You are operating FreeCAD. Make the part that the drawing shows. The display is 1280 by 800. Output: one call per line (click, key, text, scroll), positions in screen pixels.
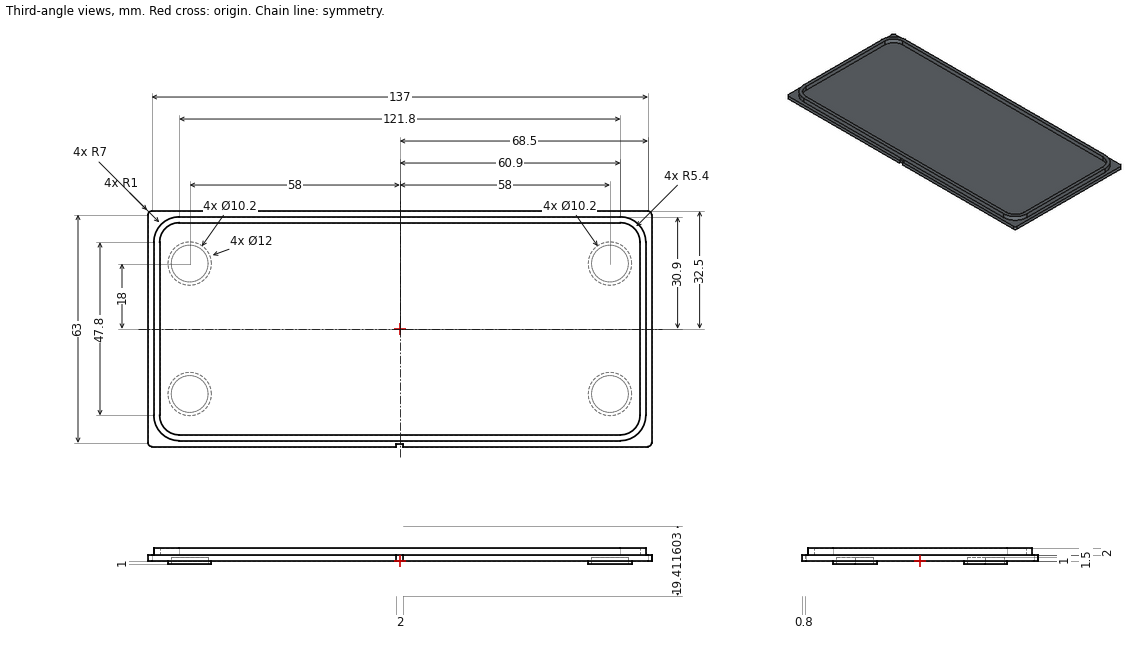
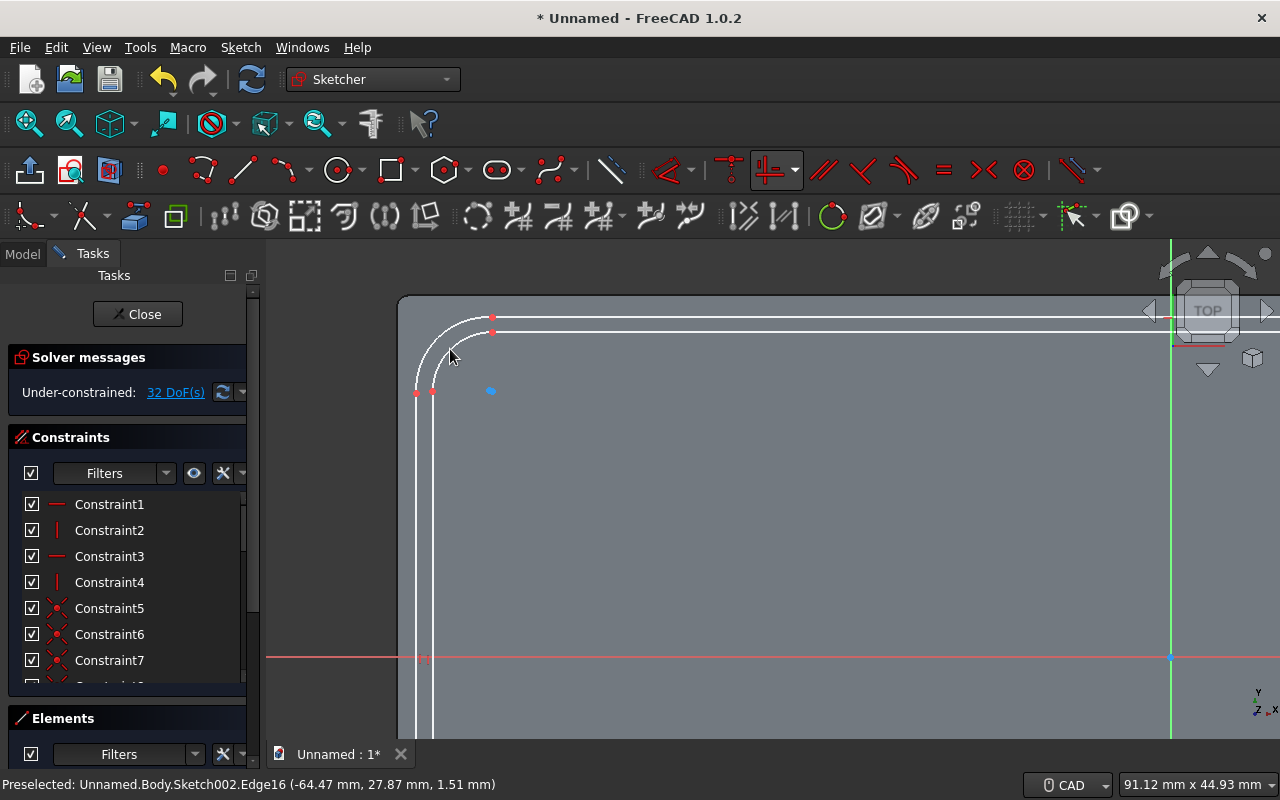
click(899, 317)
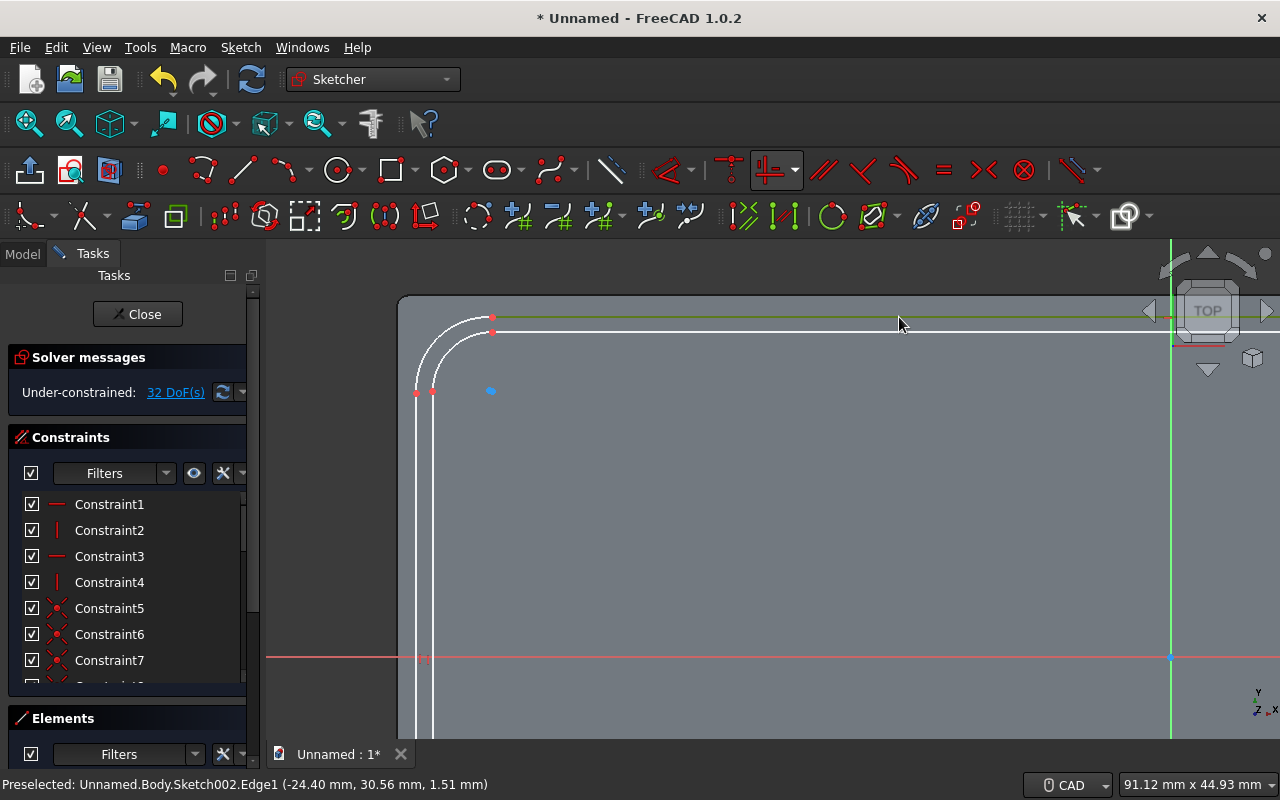
click(457, 324)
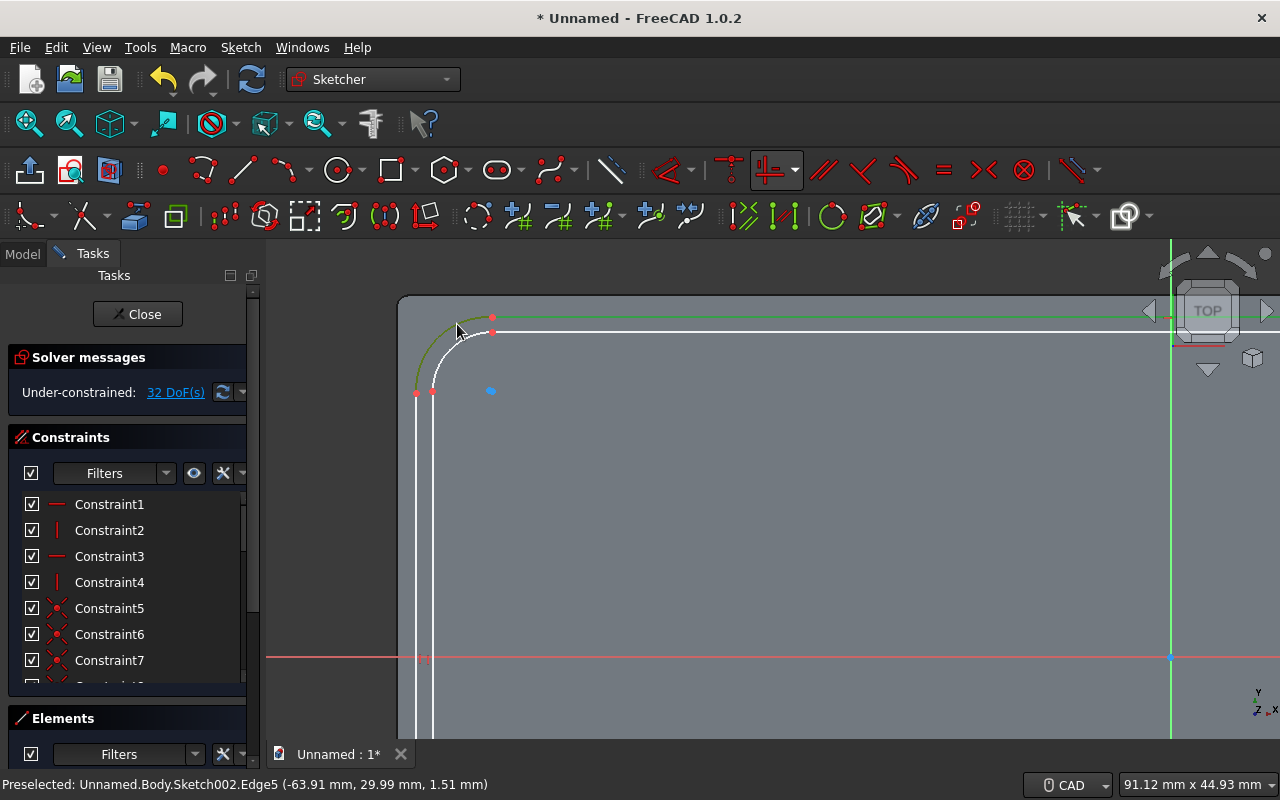
click(904, 170)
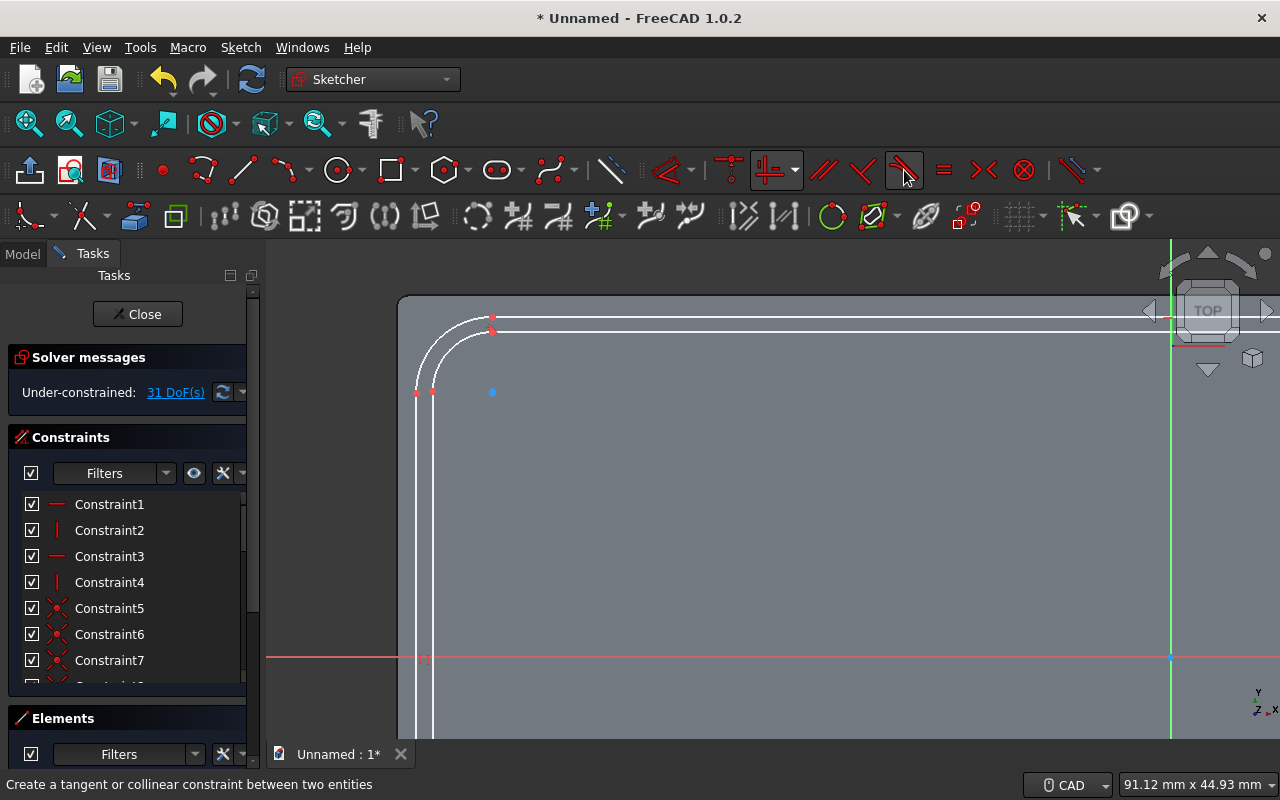
click(899, 317)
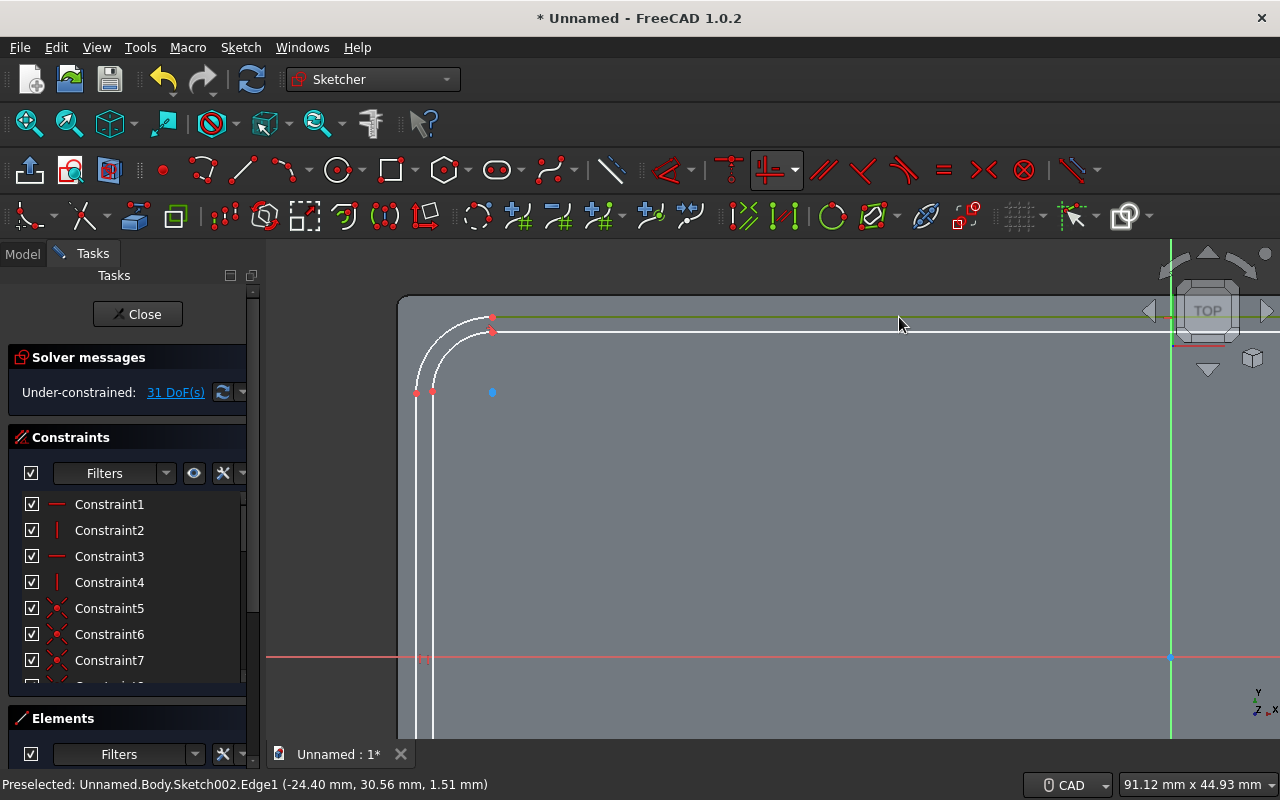
scroll(433, 391, down, 5)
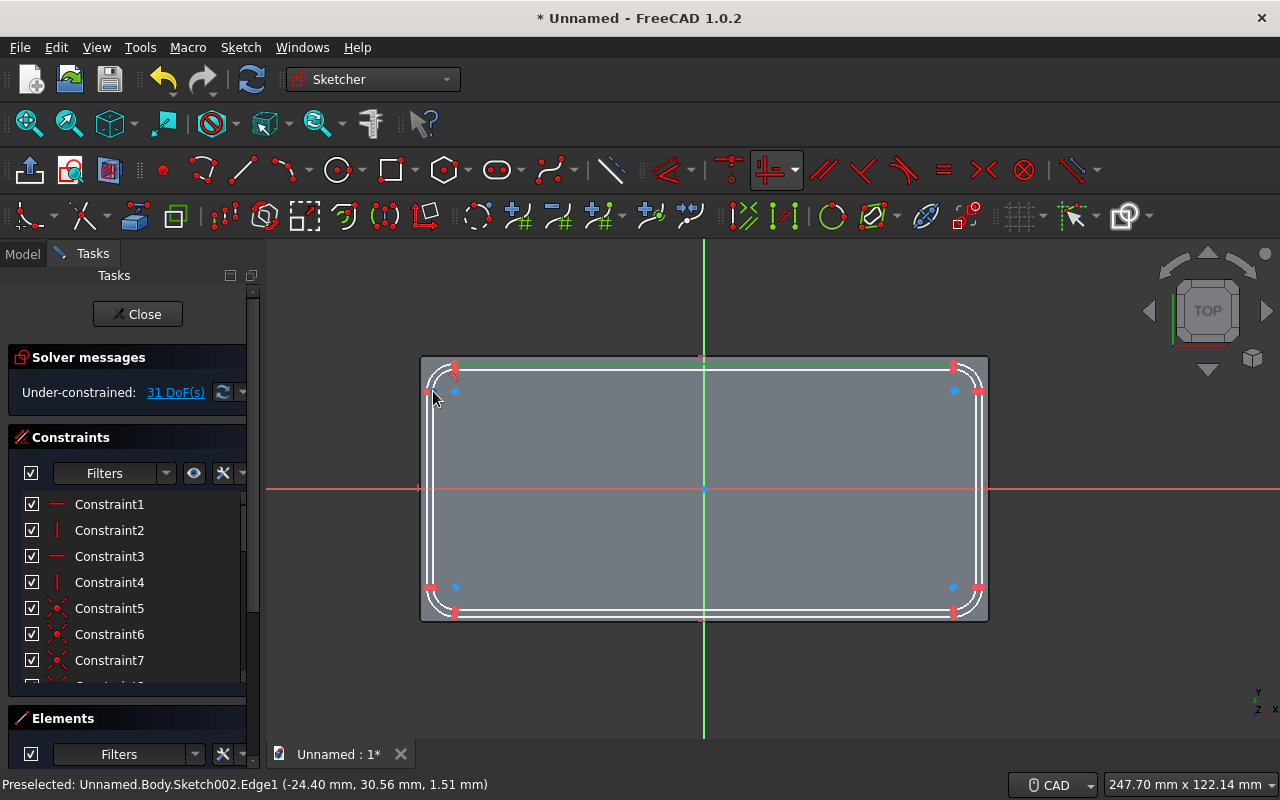
scroll(979, 379, up, 4)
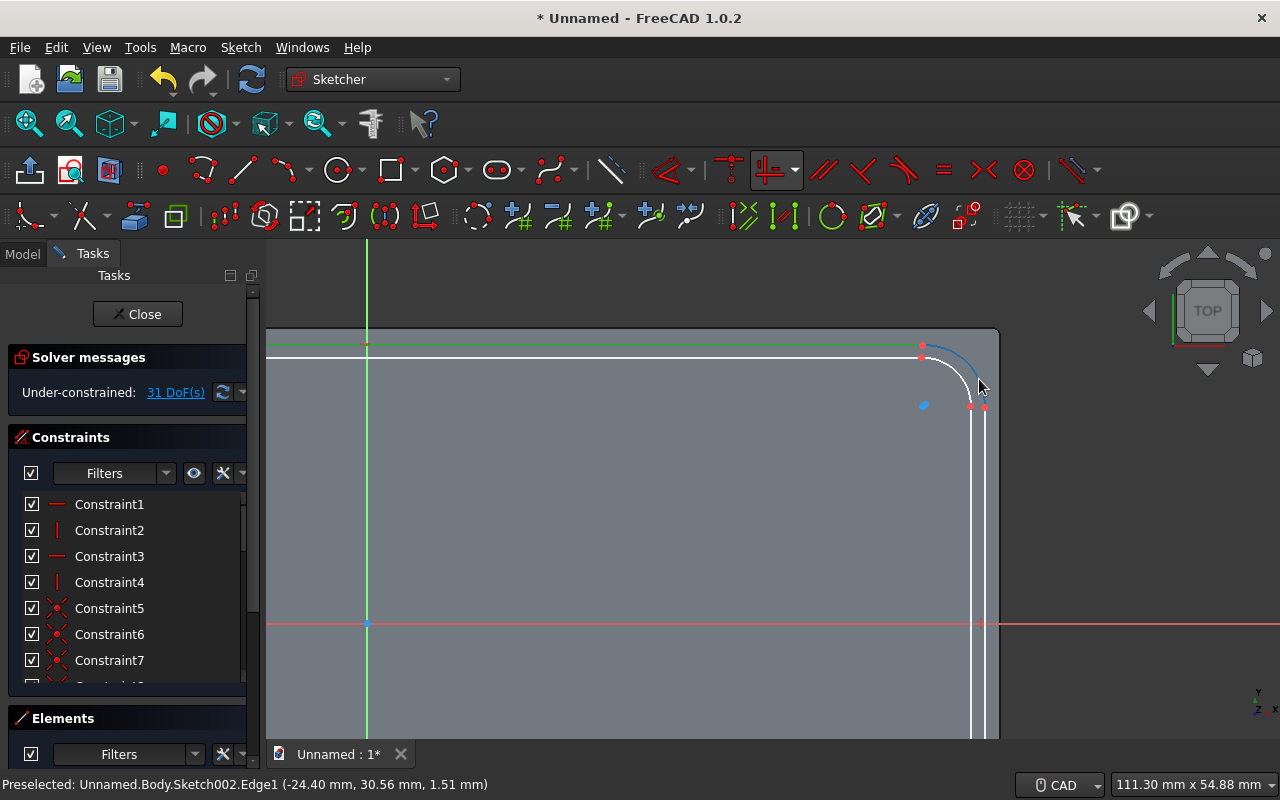
click(979, 379)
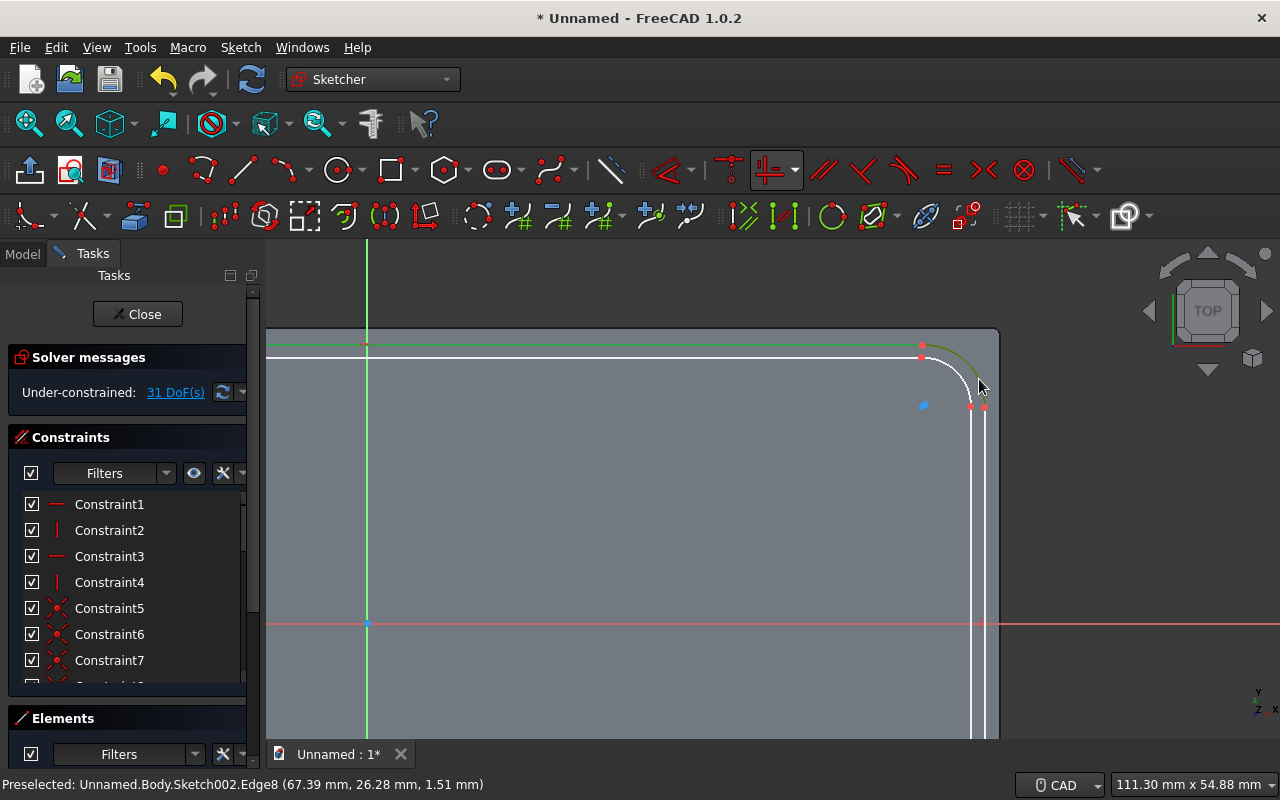
click(904, 170)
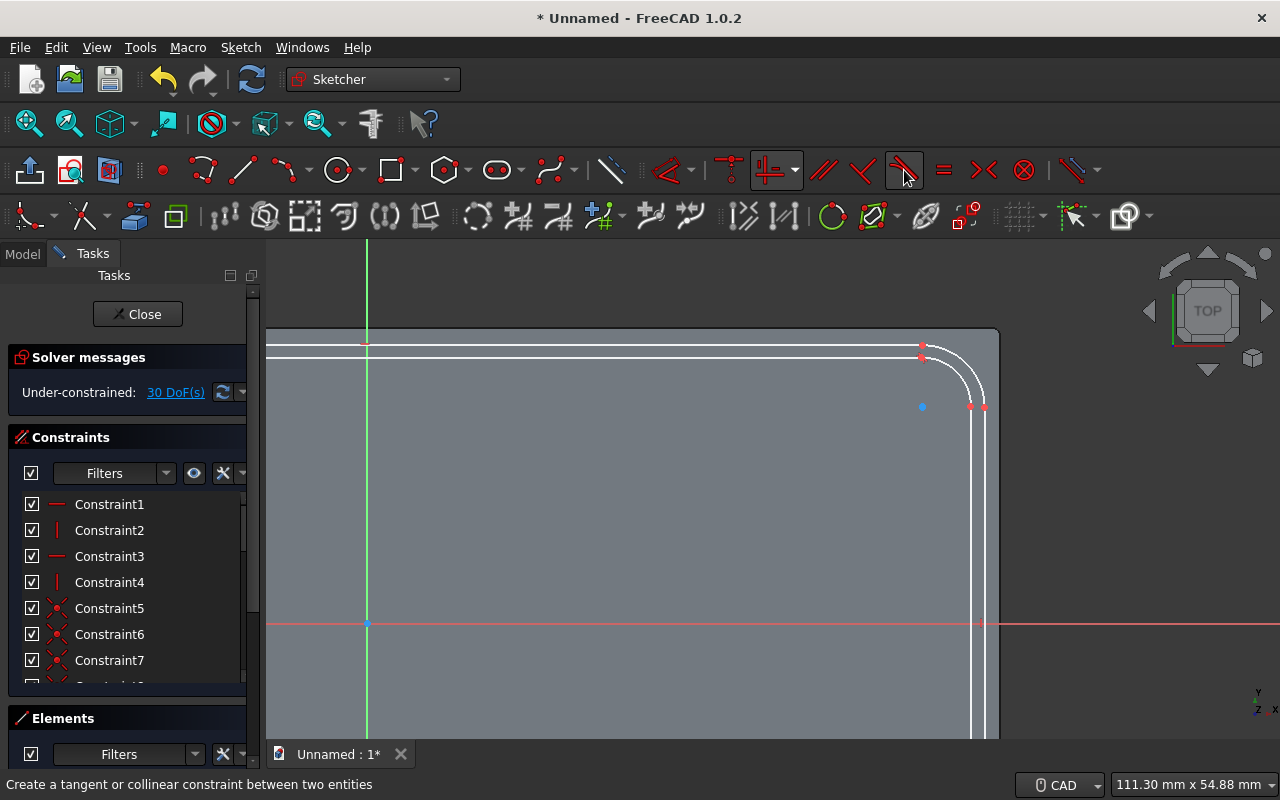
scroll(980, 379, down, 4)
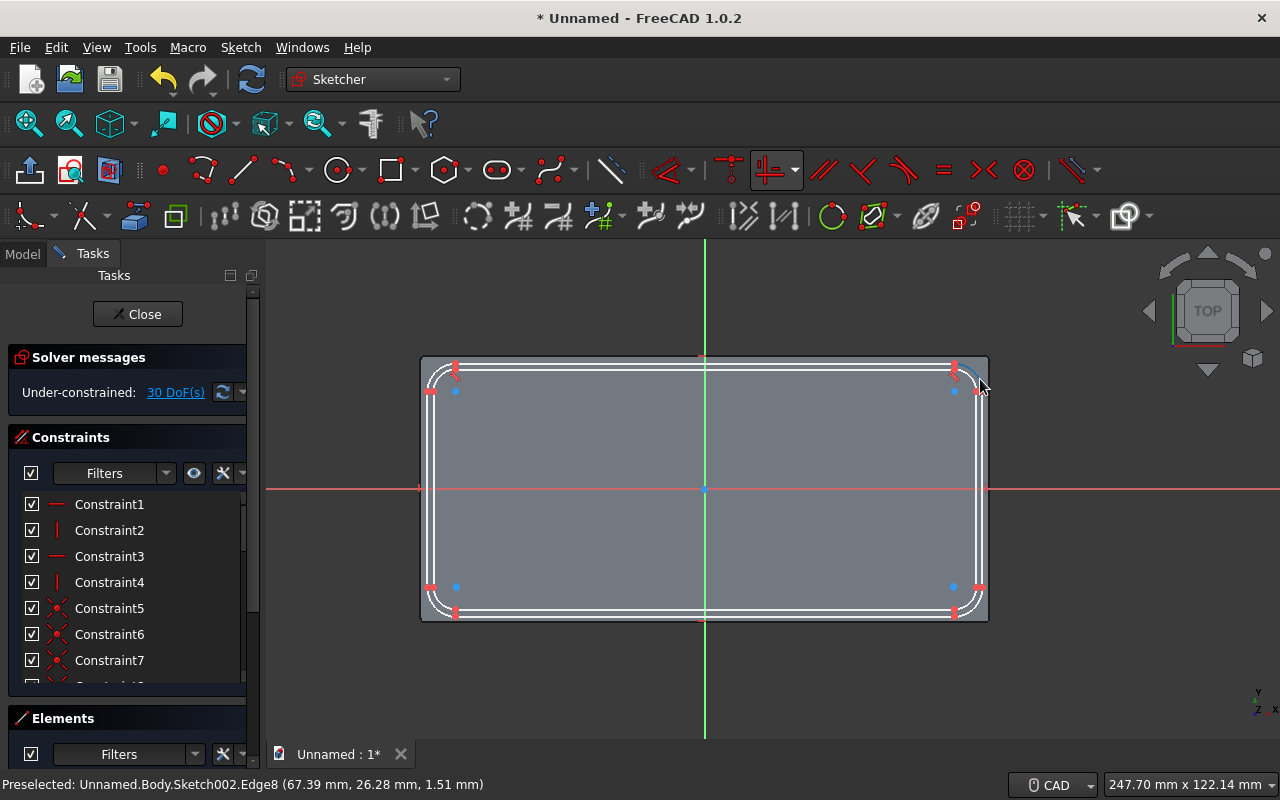
scroll(427, 451, up, 5)